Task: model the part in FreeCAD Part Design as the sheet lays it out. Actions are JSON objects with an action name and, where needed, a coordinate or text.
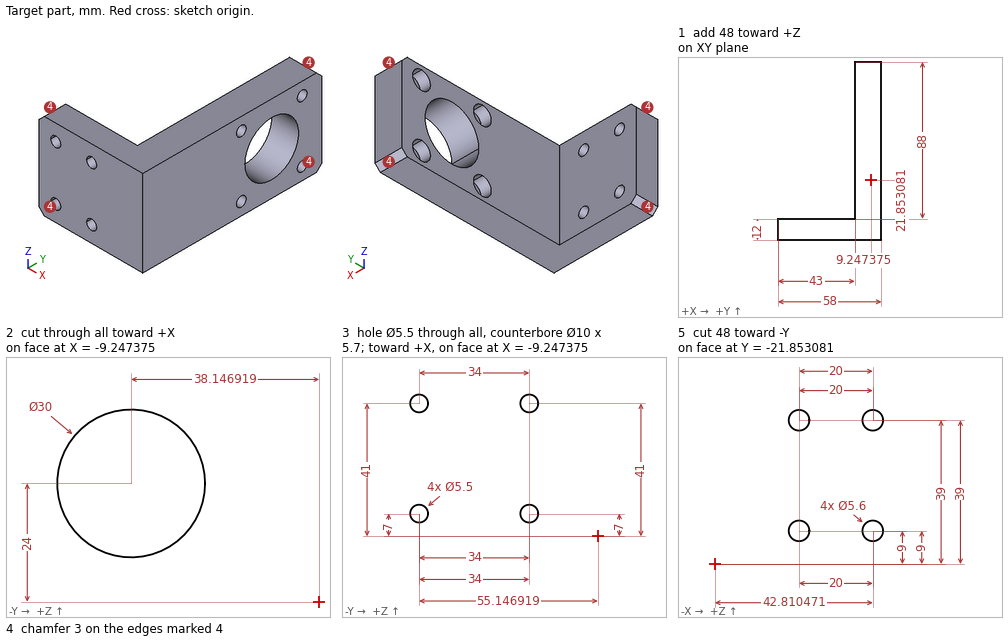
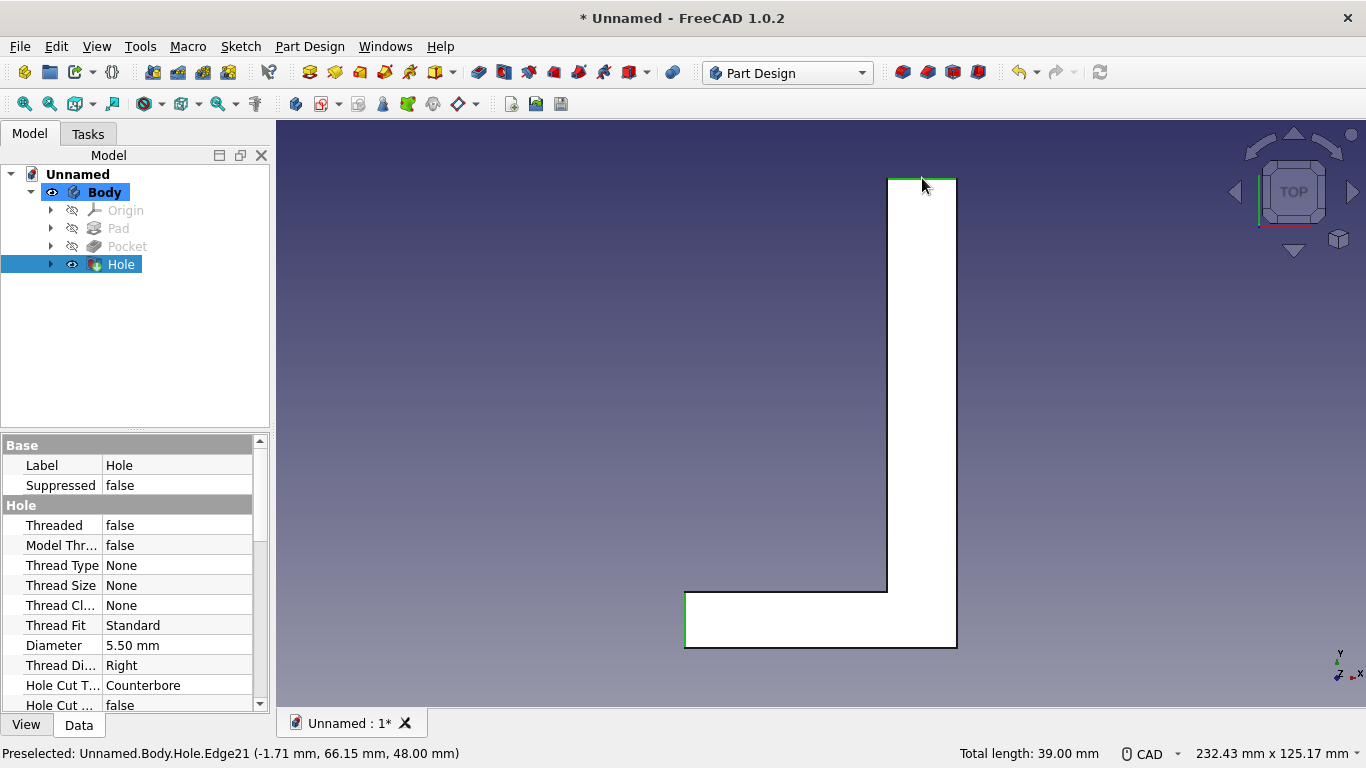
{"action": "key", "text": "1"}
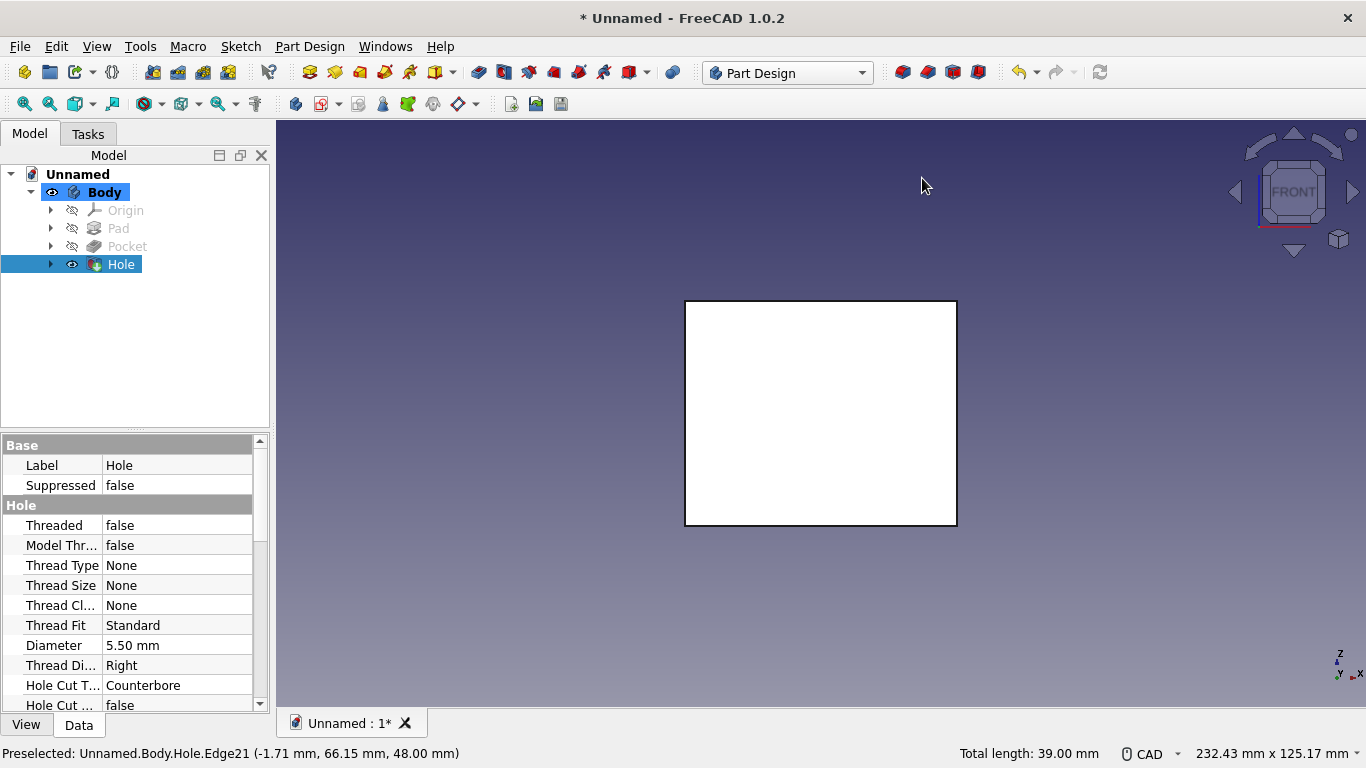
{"action": "left_click", "coordinate": [25, 104]}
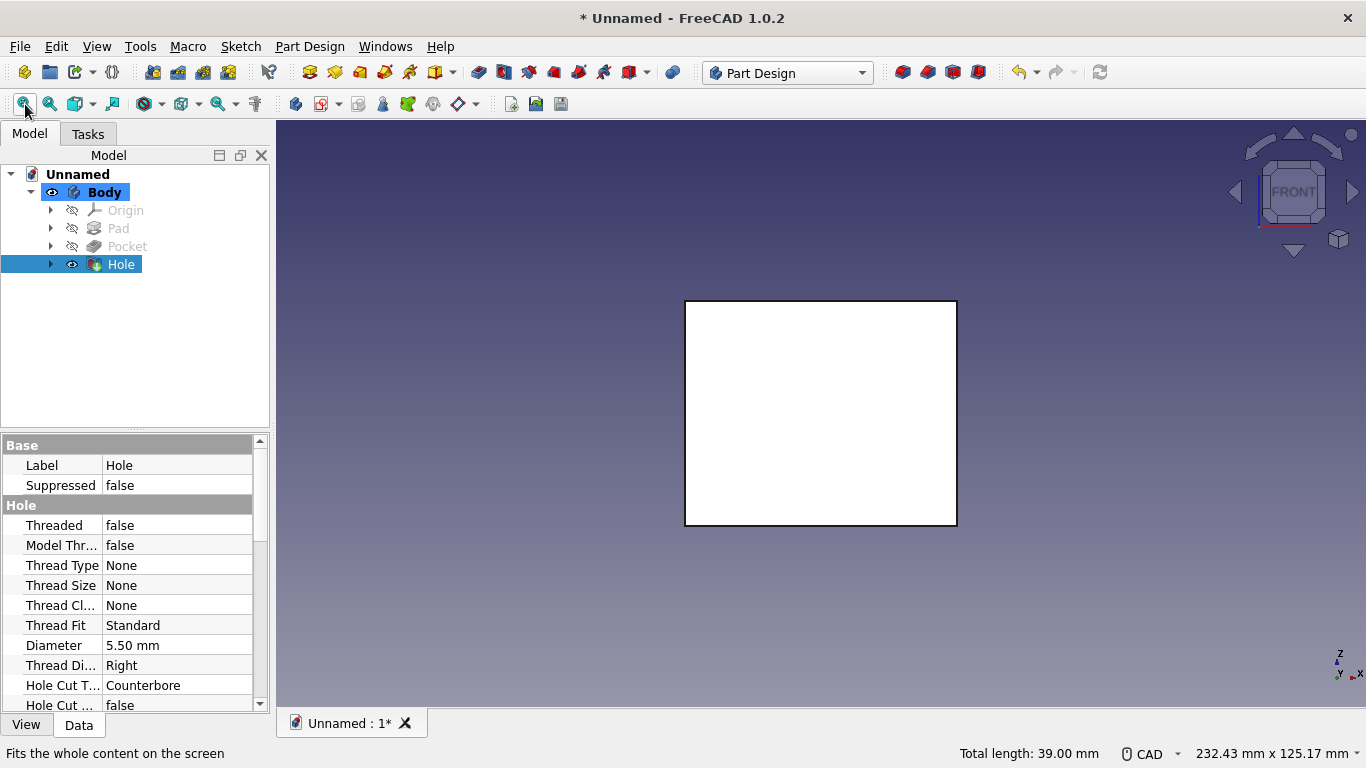
{"action": "key", "text": "3"}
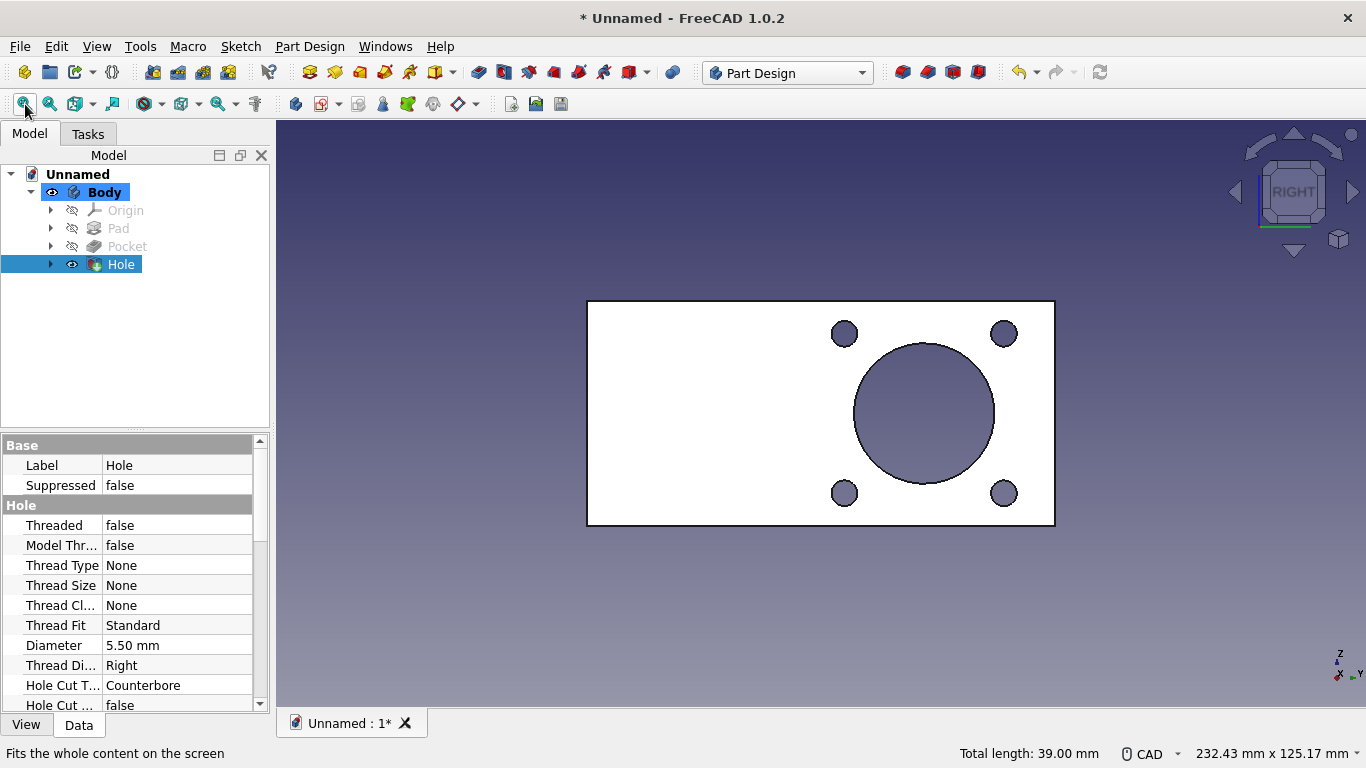
{"action": "key", "text": "v f"}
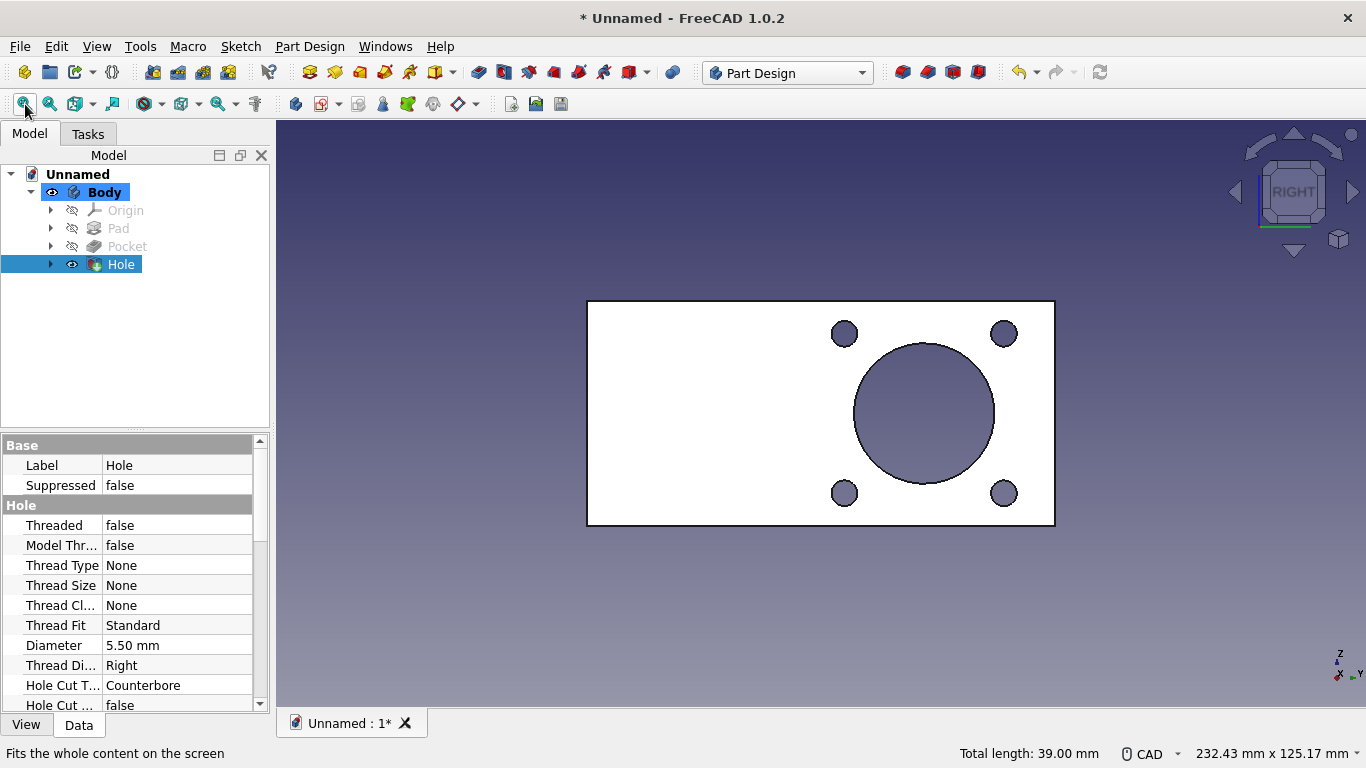
{"action": "key", "text": "5"}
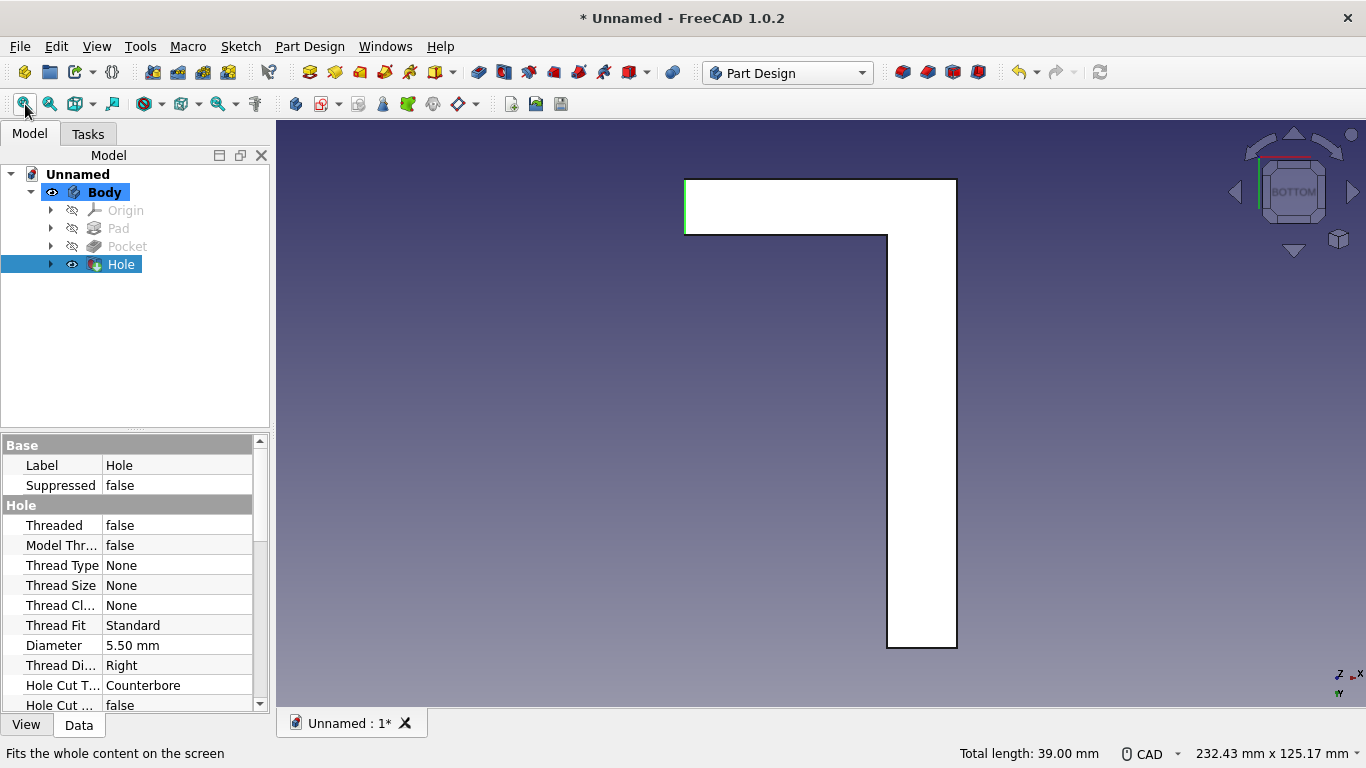
{"action": "left_click", "coordinate": [922, 647], "text": "ctrl"}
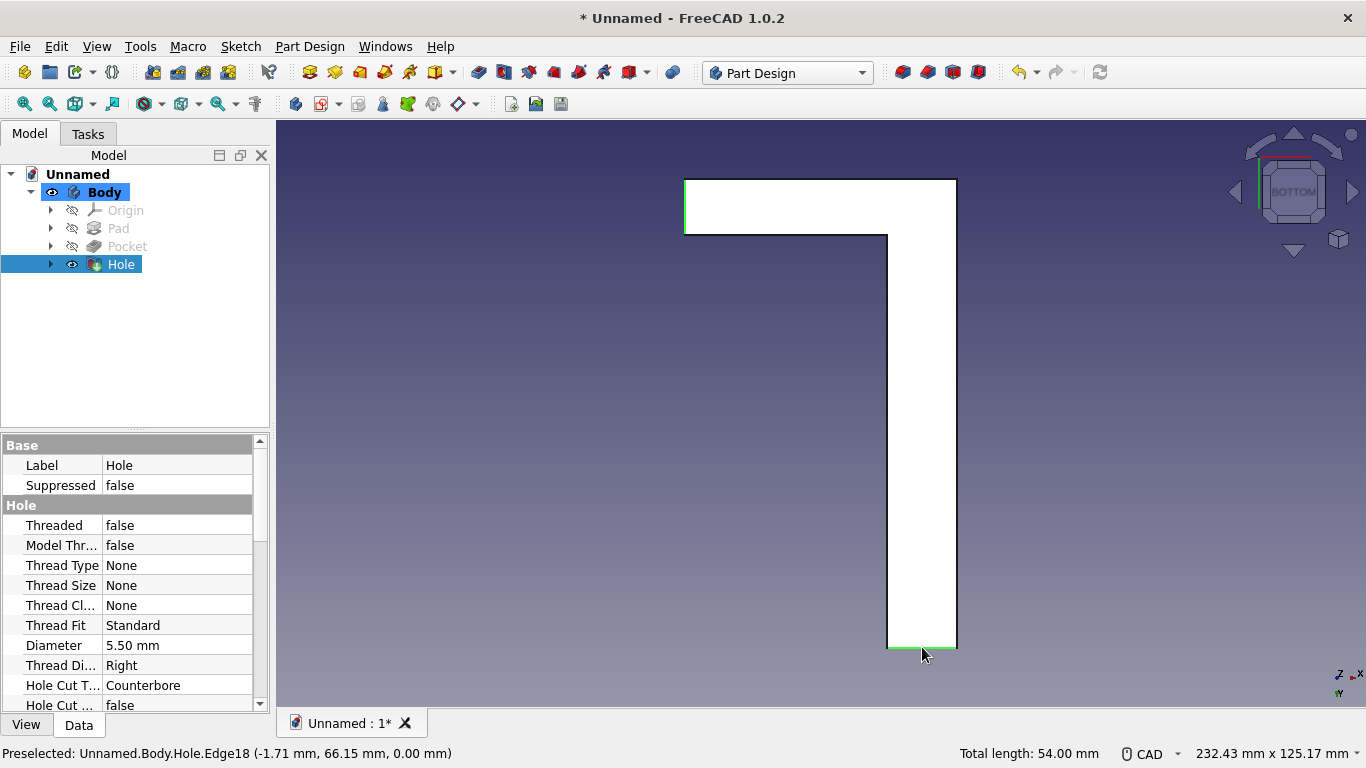
{"action": "left_click", "coordinate": [928, 72]}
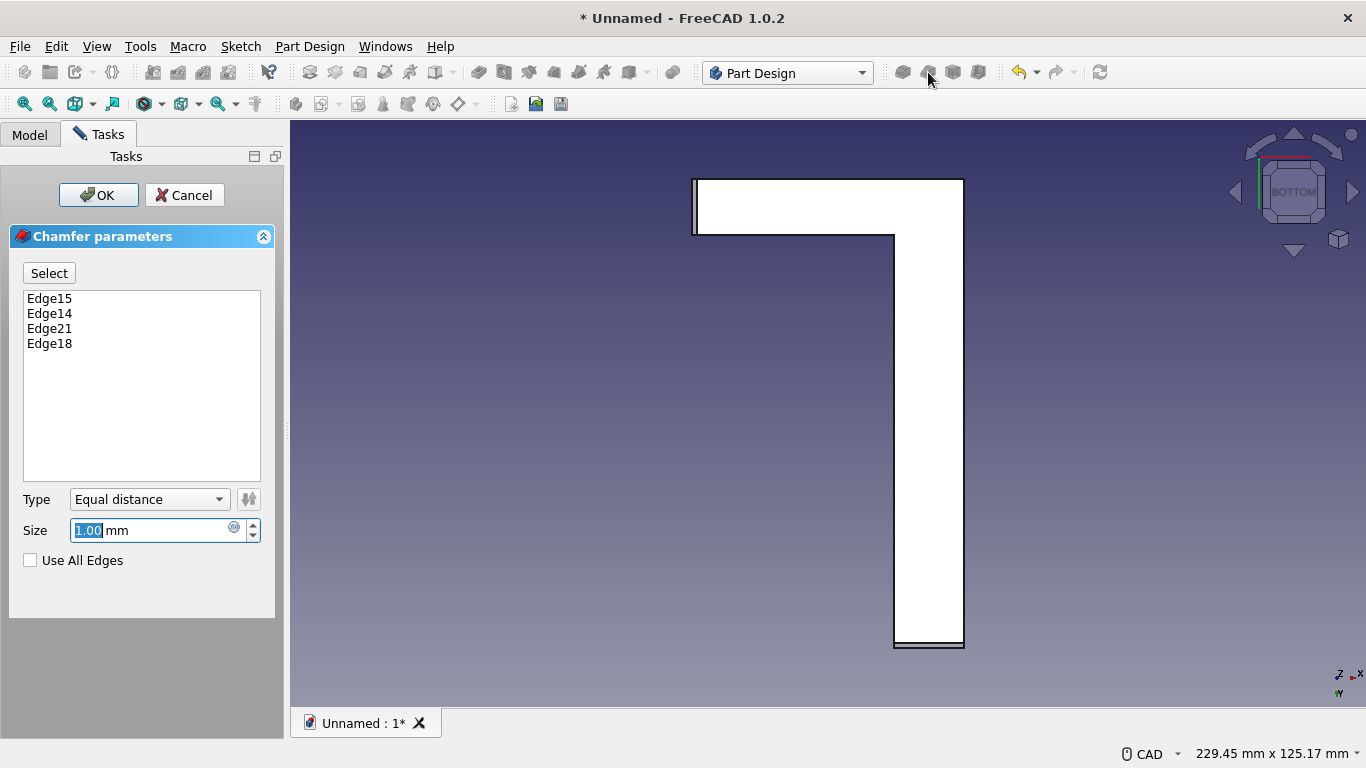
{"action": "type", "text": "3"}
{"action": "key", "text": "Tab"}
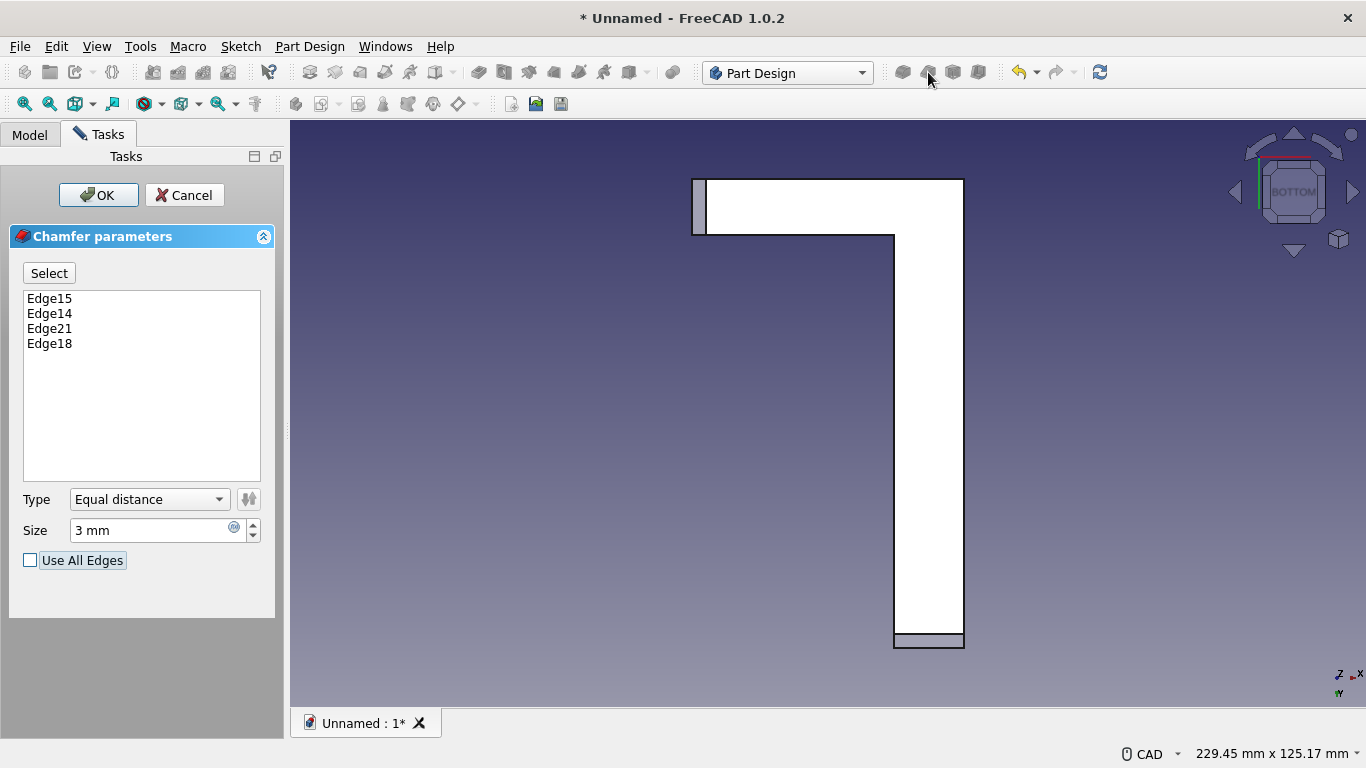
{"action": "left_click", "coordinate": [99, 195]}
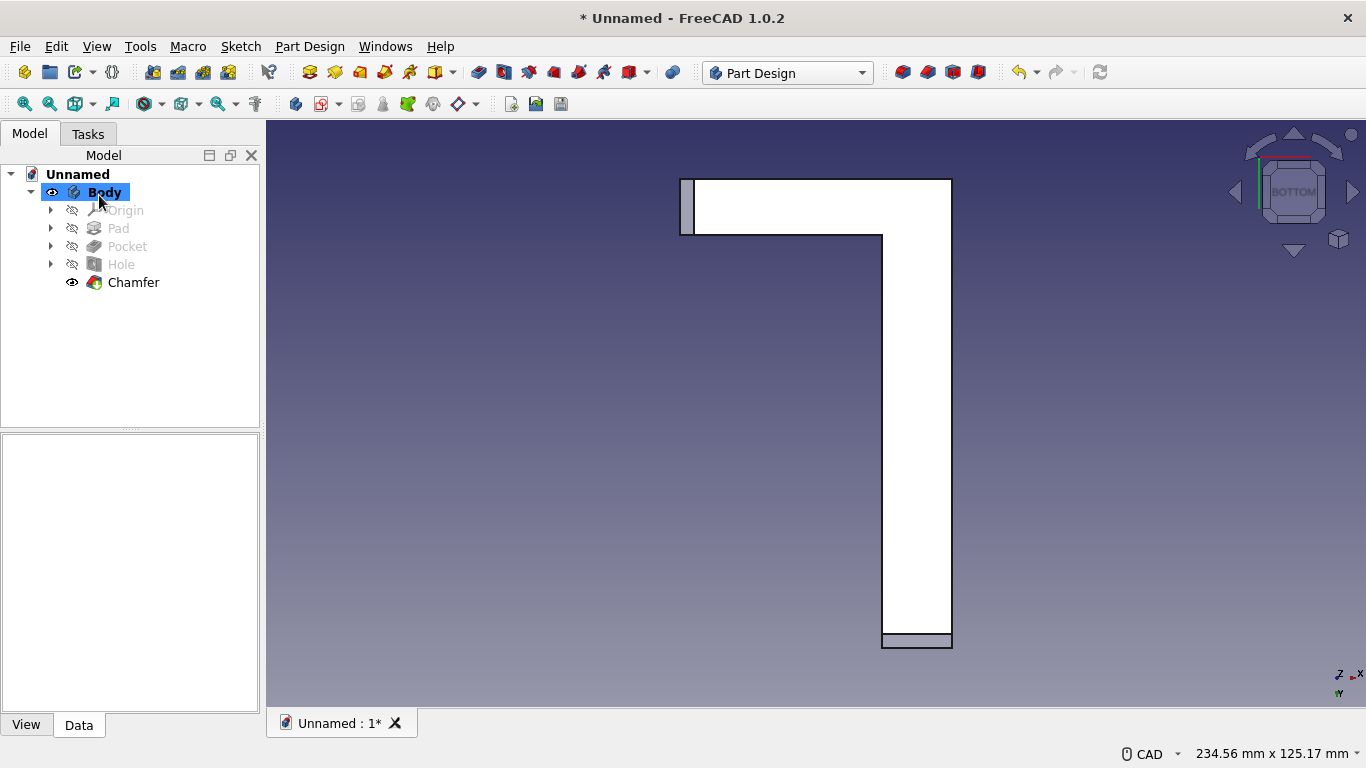
{"action": "key", "text": "4"}